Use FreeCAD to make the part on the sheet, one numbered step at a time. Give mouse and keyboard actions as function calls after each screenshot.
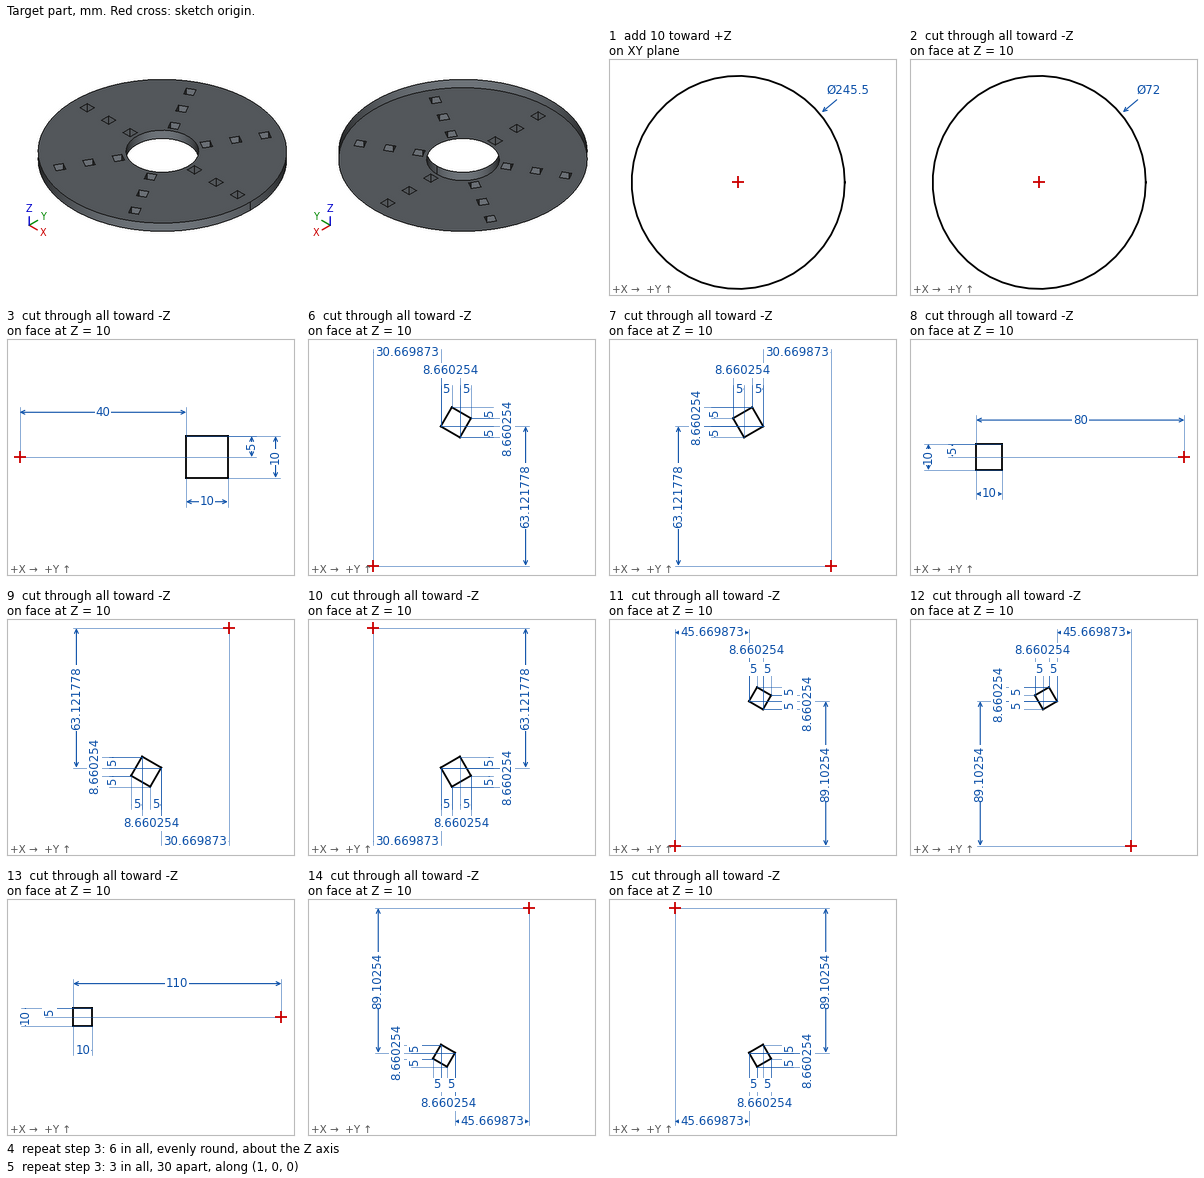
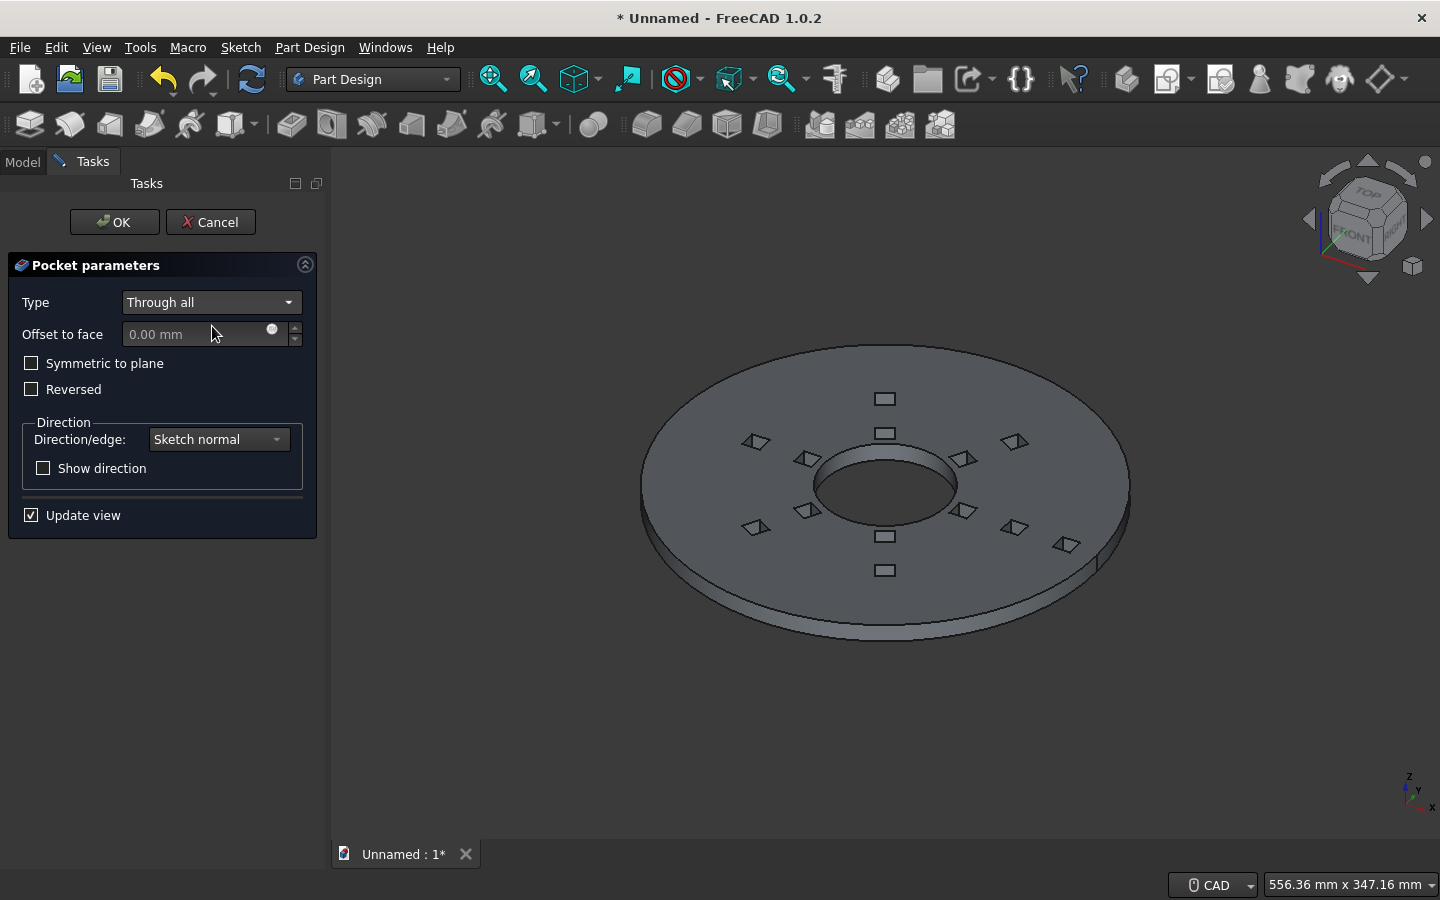
click(115, 222)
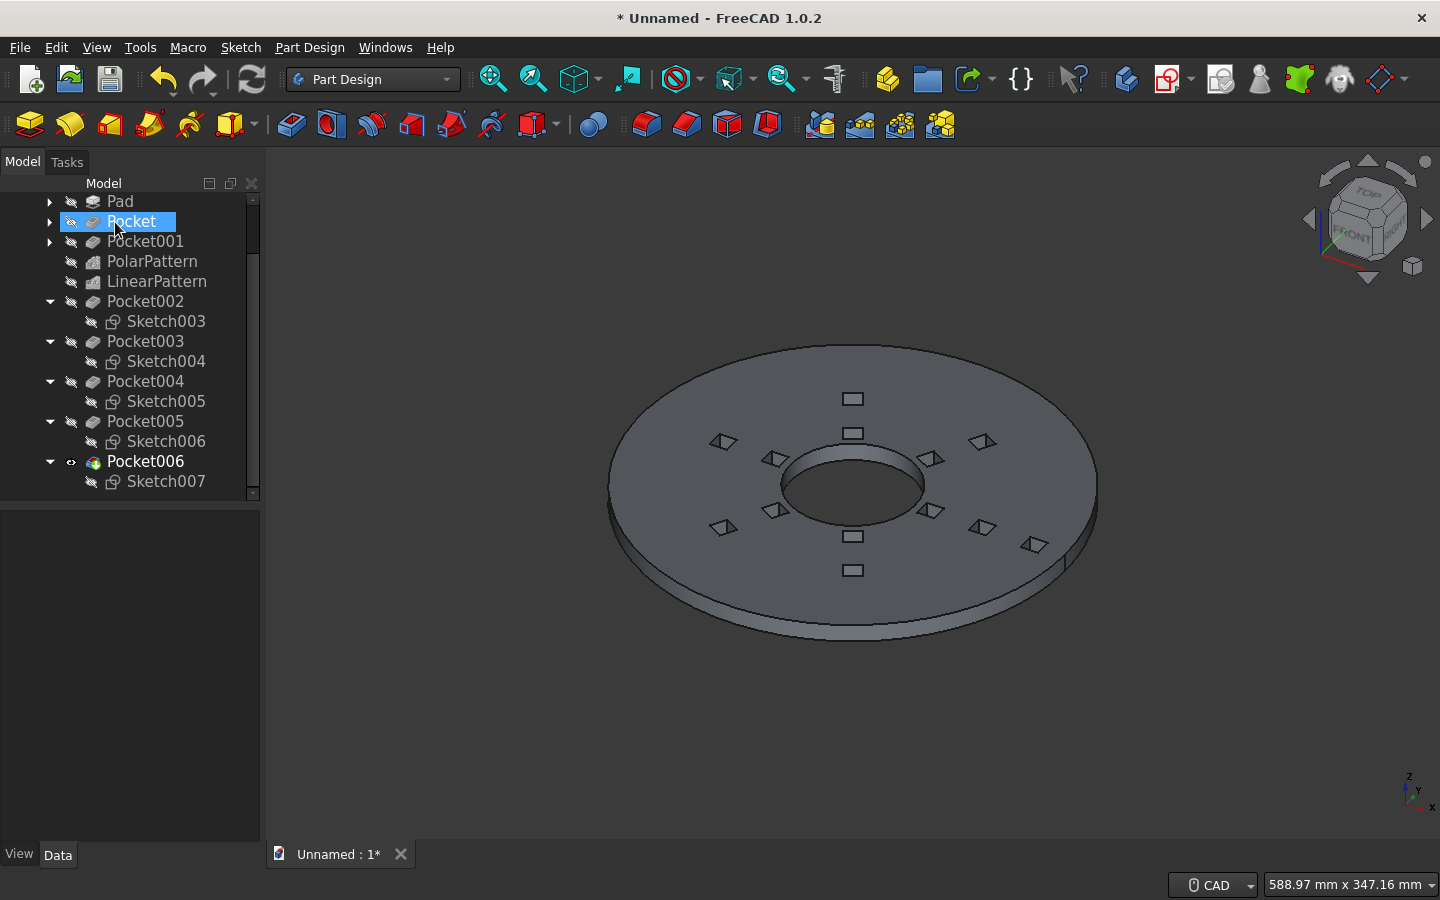
click(923, 414)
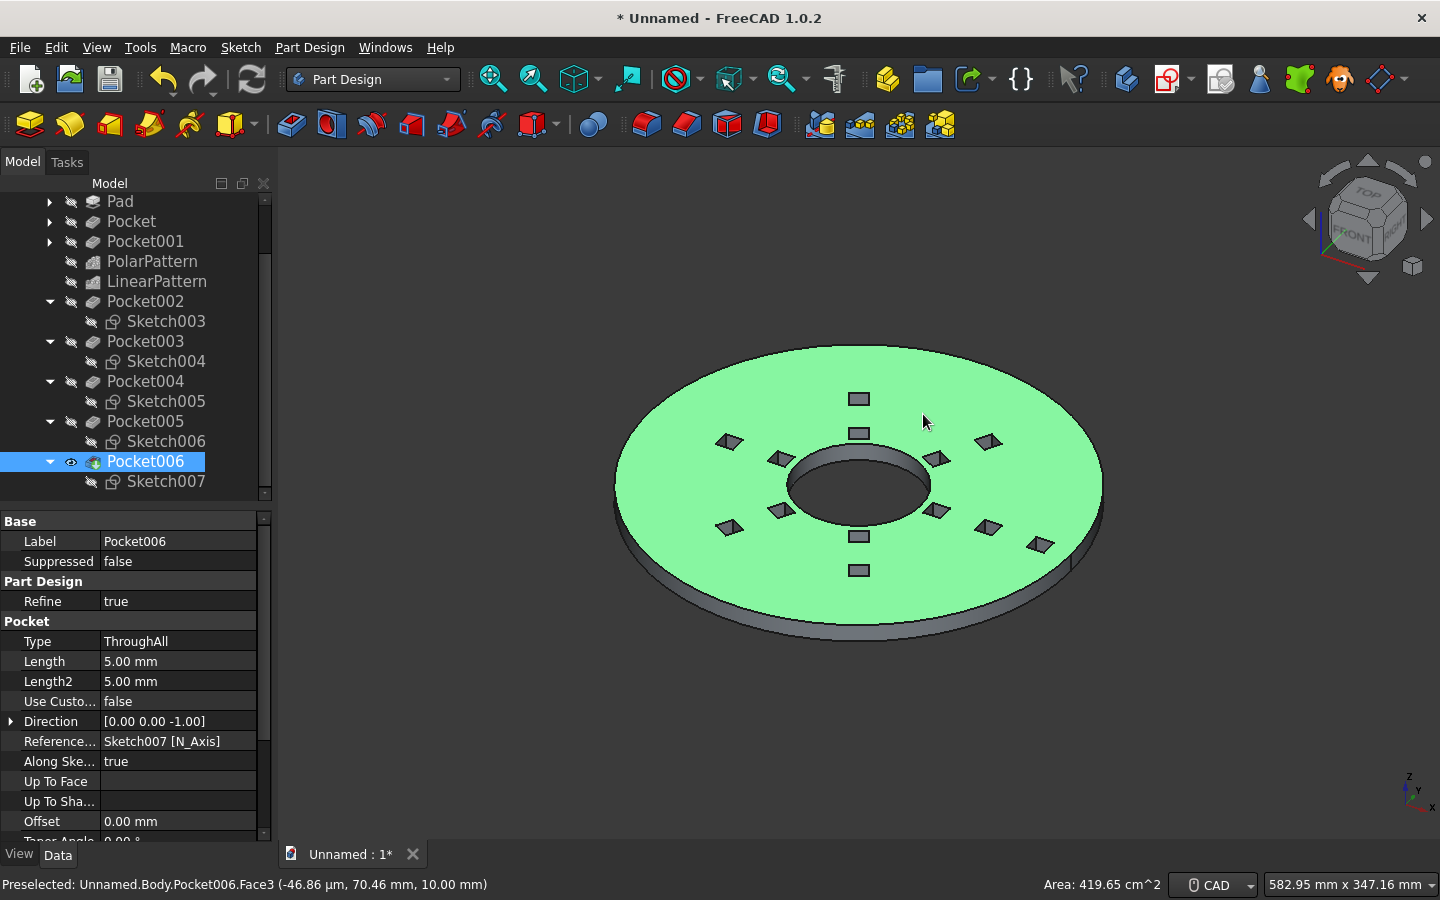
click(1168, 80)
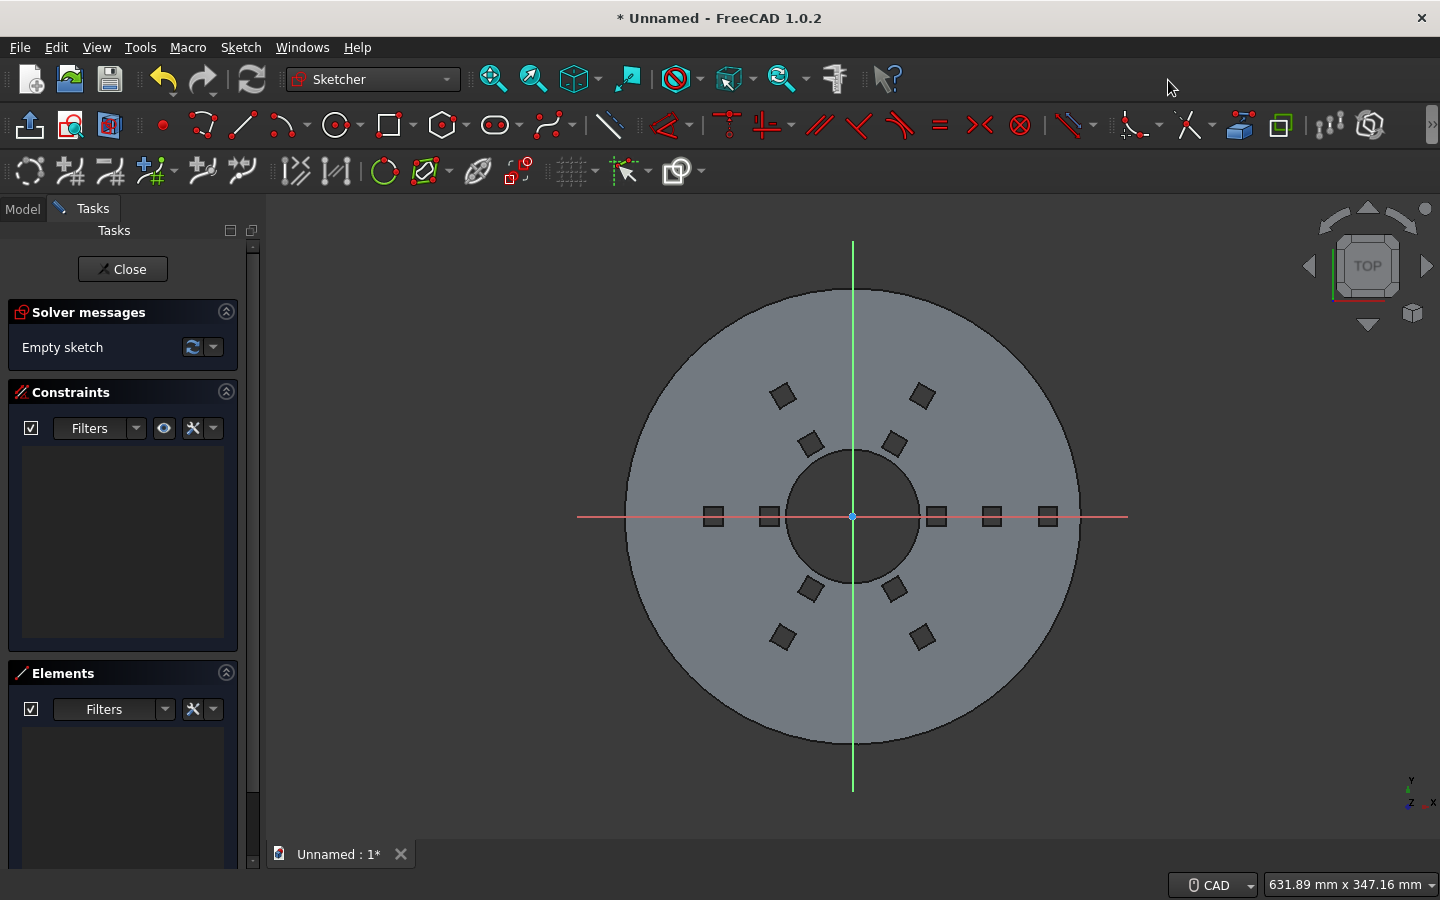
scroll(961, 337, up, 14)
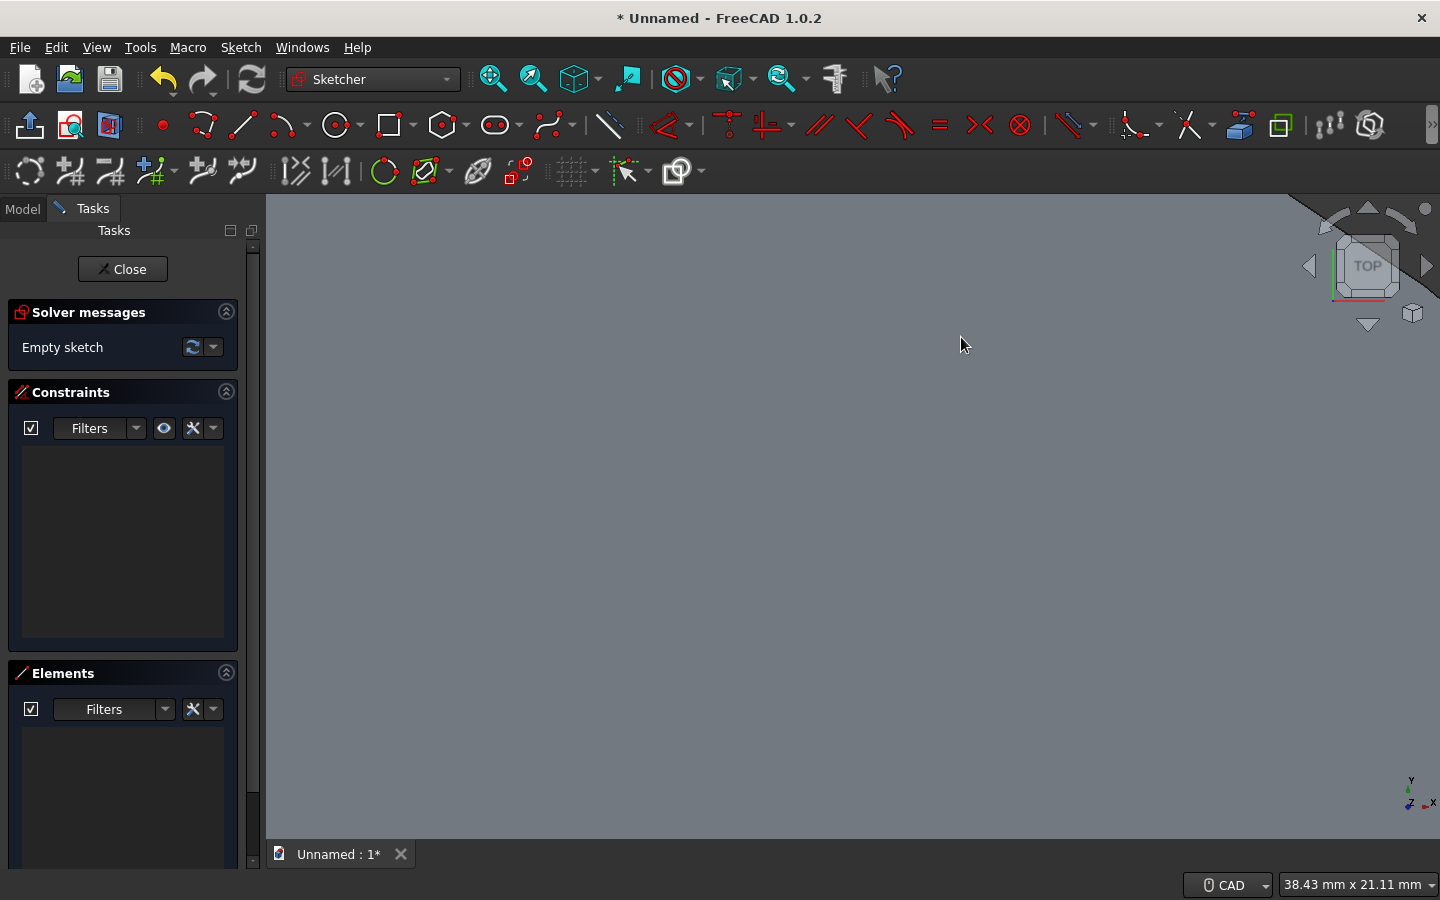
key(g)
key(m)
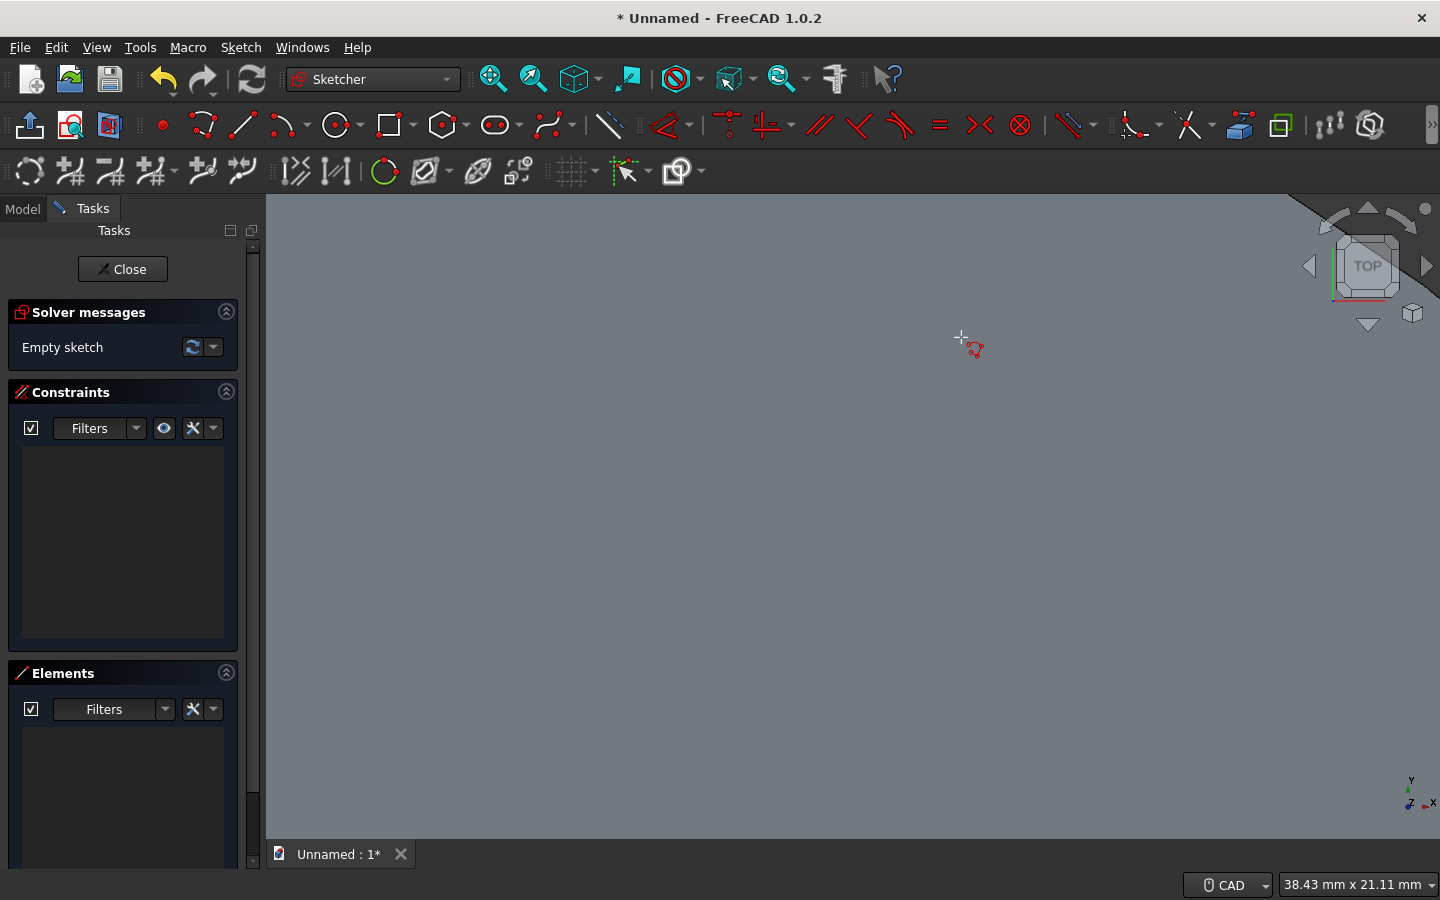
click(569, 563)
click(833, 716)
click(986, 451)
click(721, 298)
click(569, 564)
key(Escape)
key(Escape)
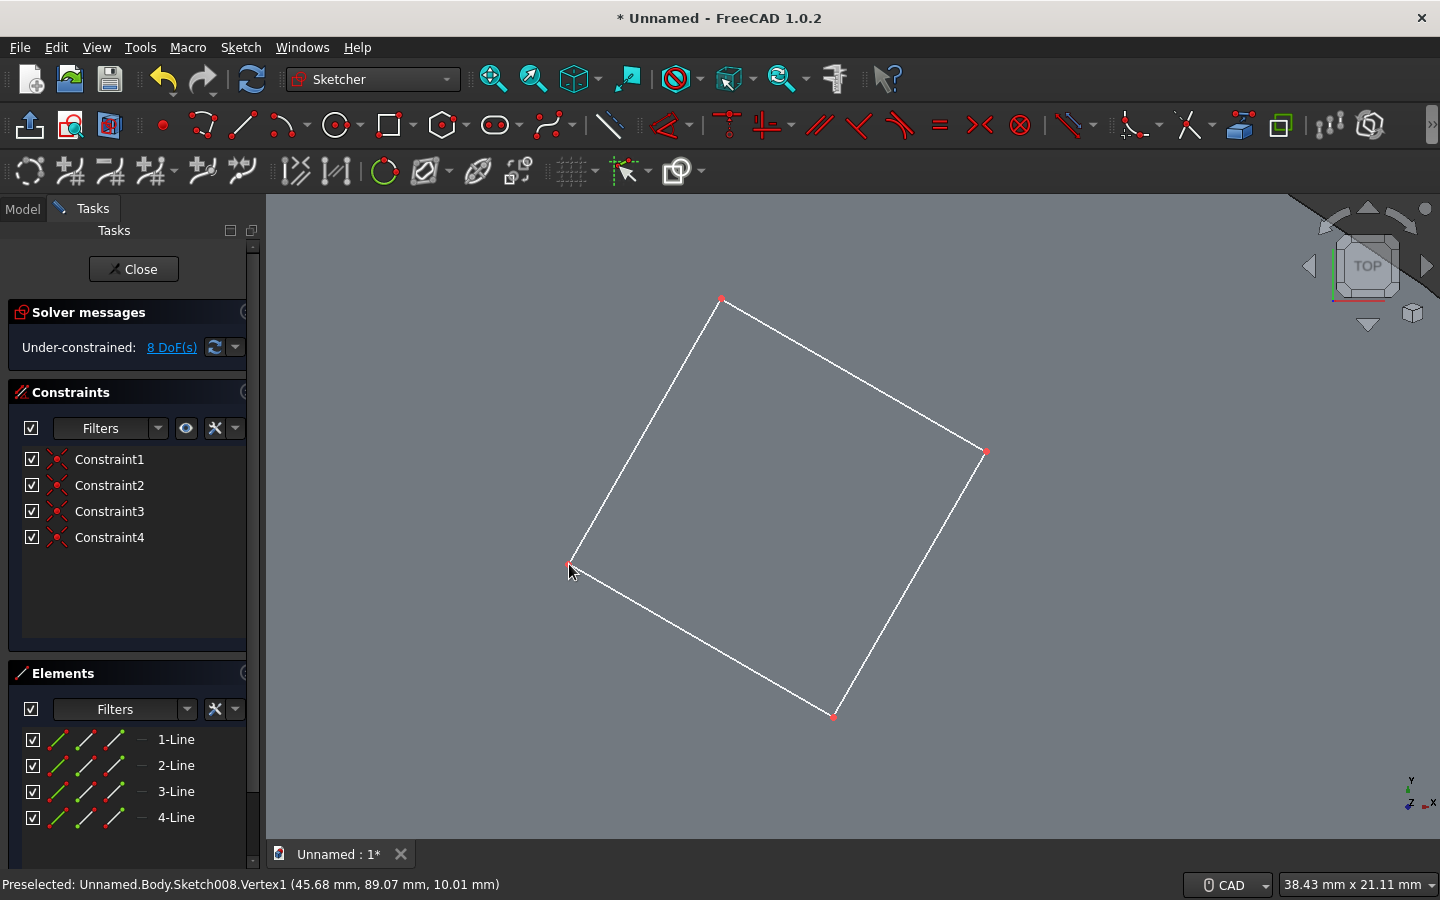
key(d)